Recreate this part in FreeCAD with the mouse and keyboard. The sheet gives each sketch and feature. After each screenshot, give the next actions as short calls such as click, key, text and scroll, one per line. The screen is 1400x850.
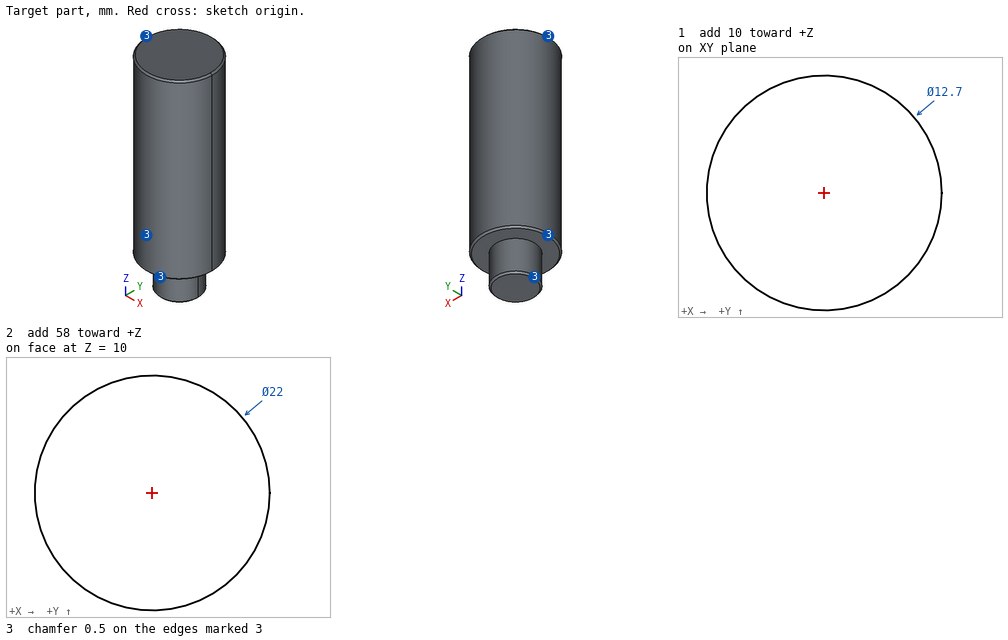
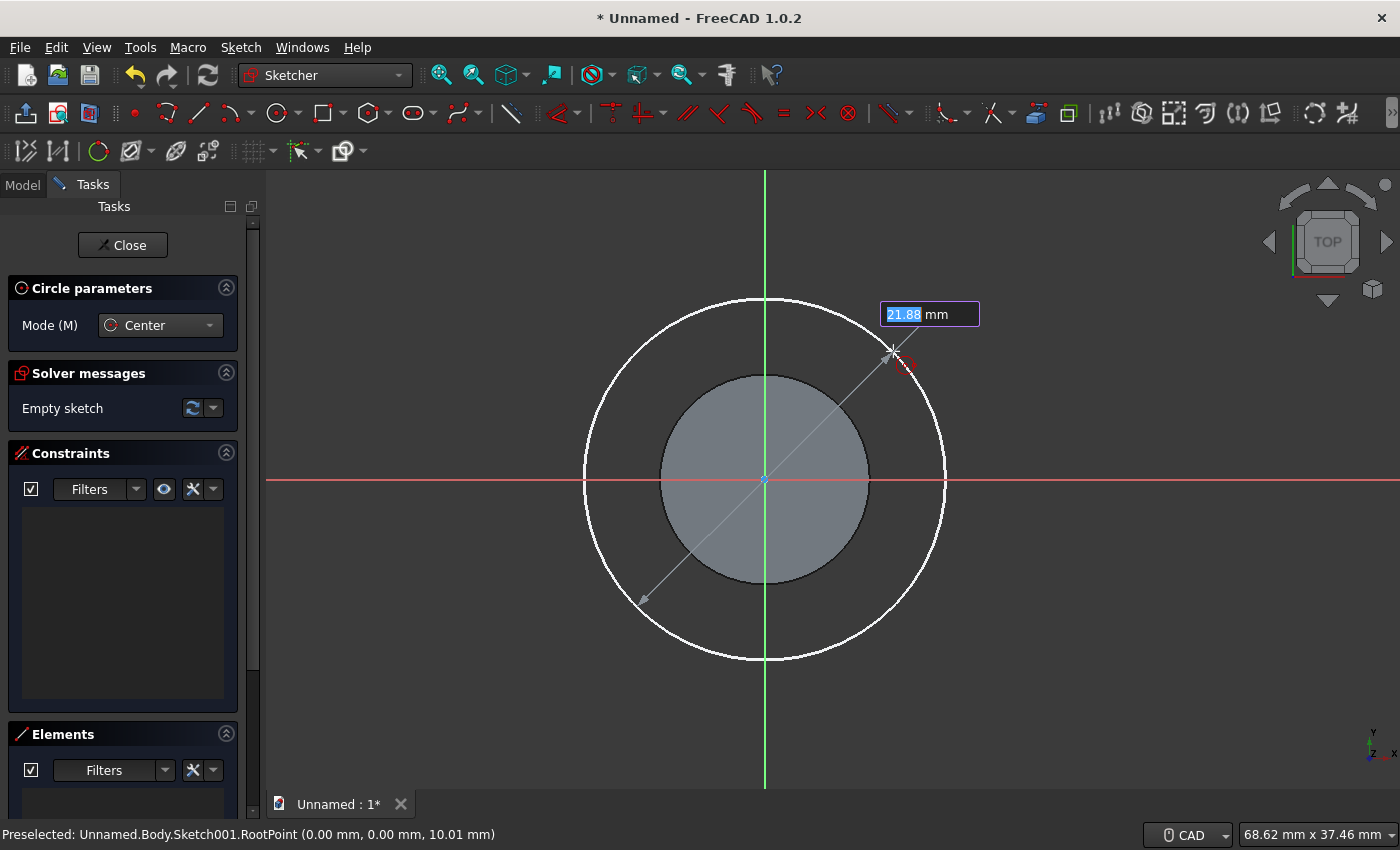
text(22)
key(Return)
key(Escape)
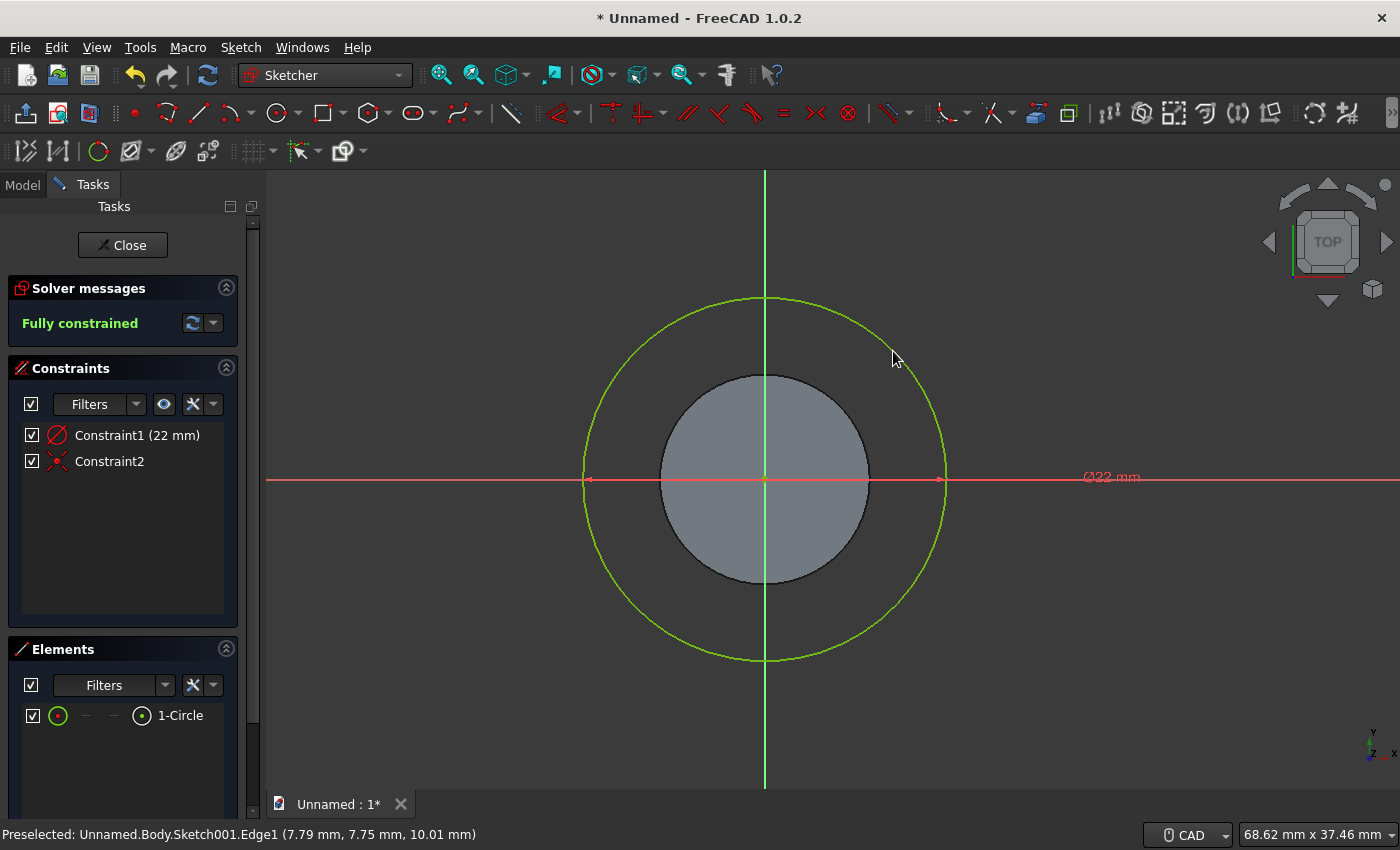
click(123, 245)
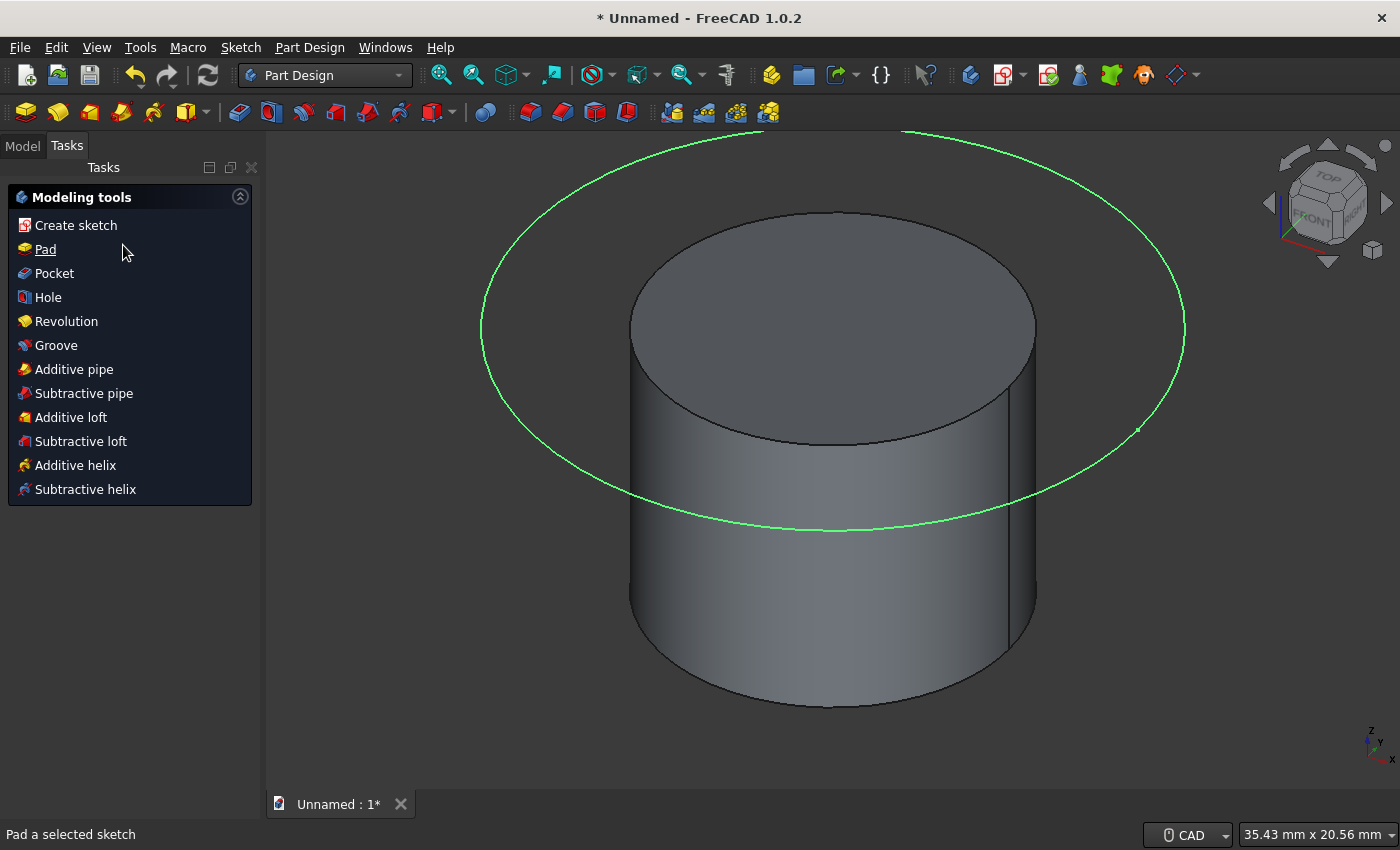
click(26, 112)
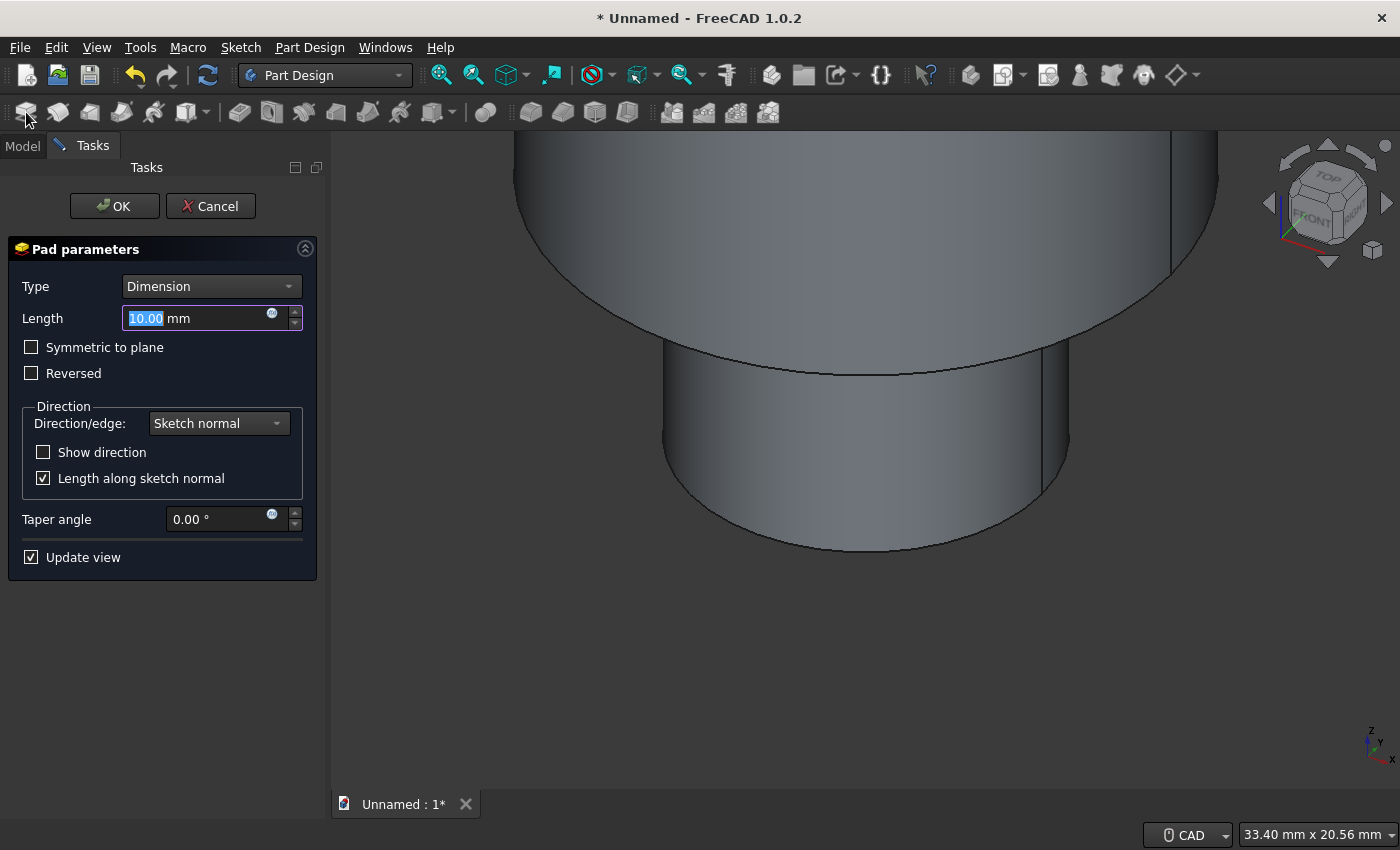
text(58)
key(Tab)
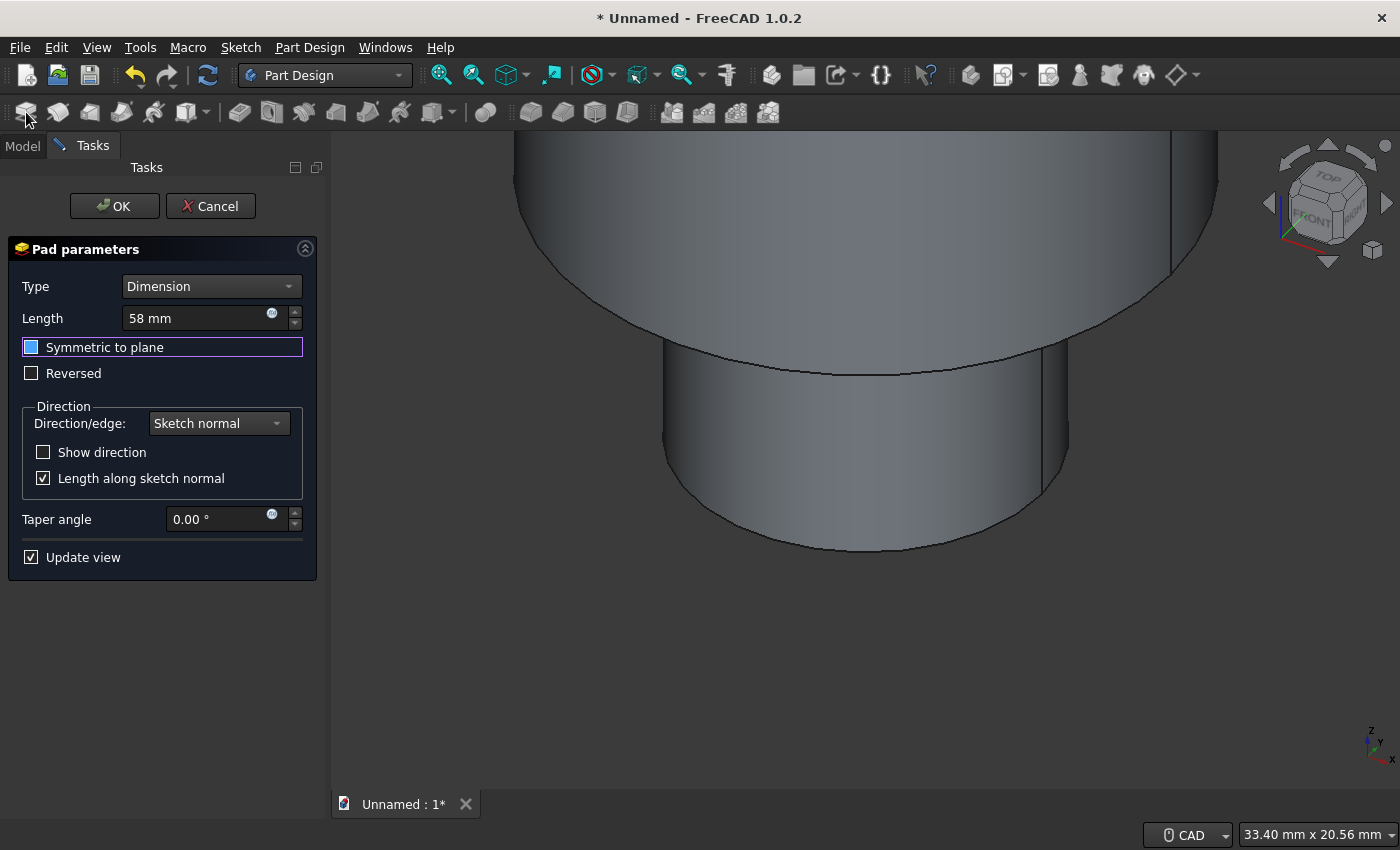
click(115, 206)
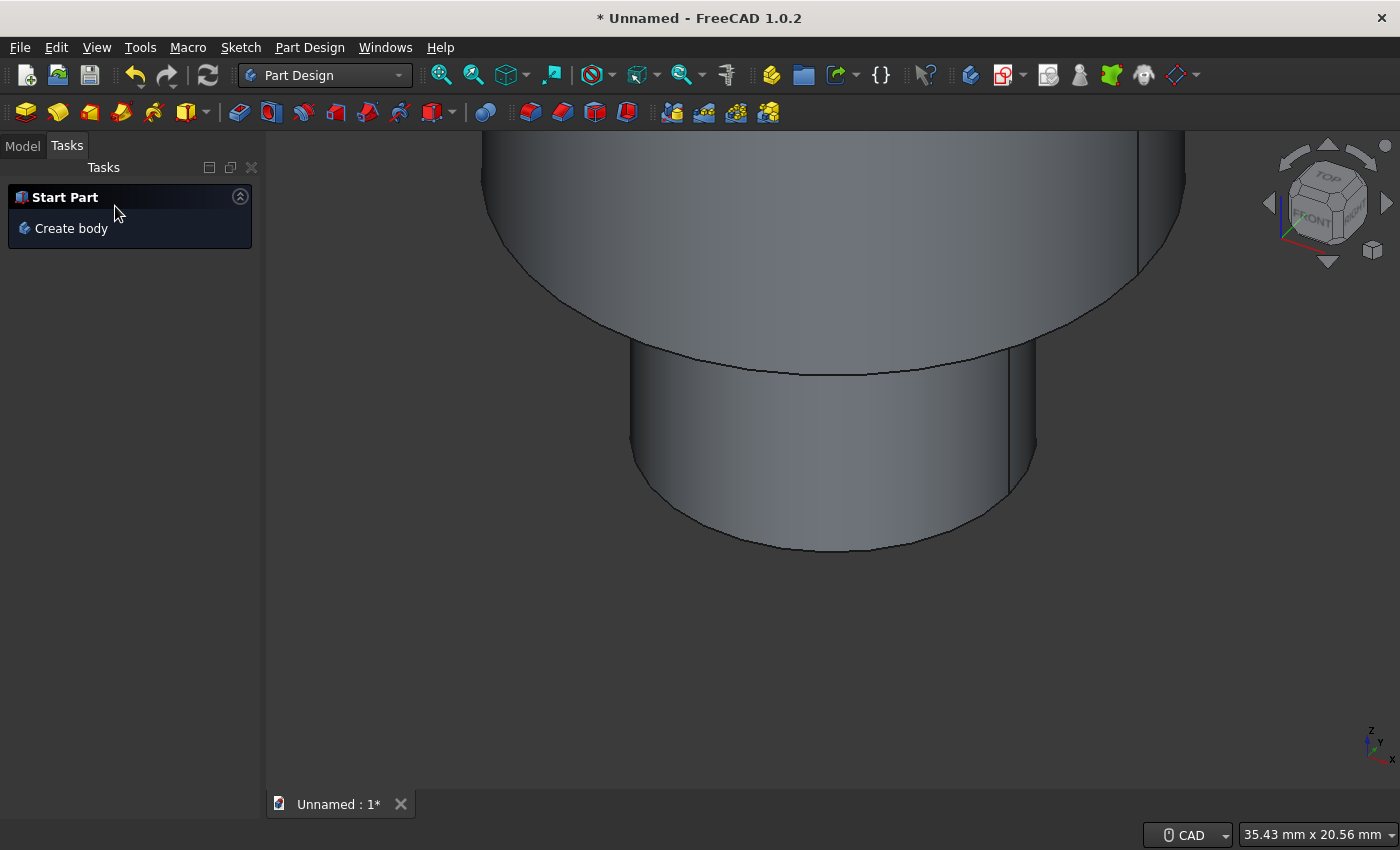
click(442, 76)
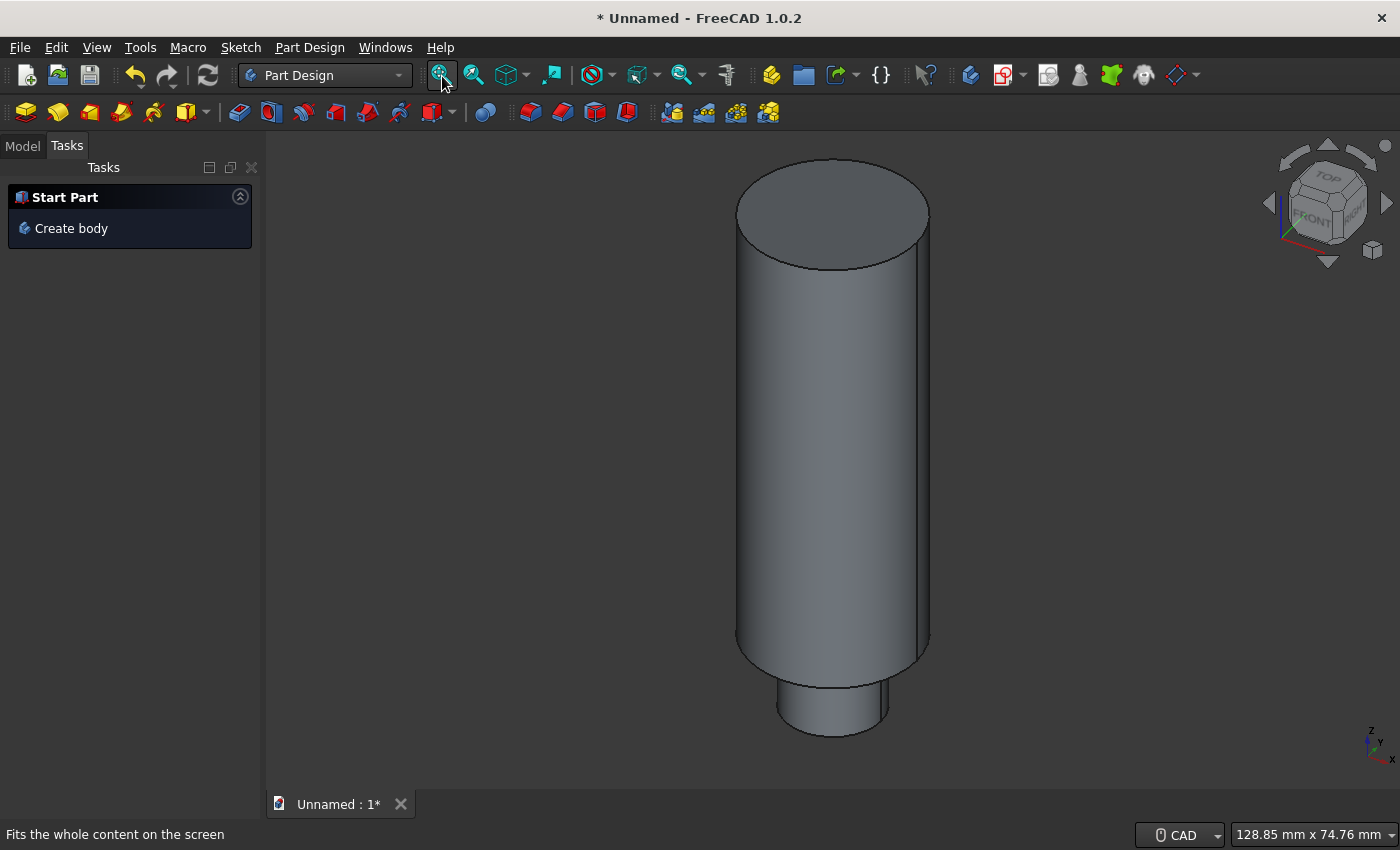
click(737, 220)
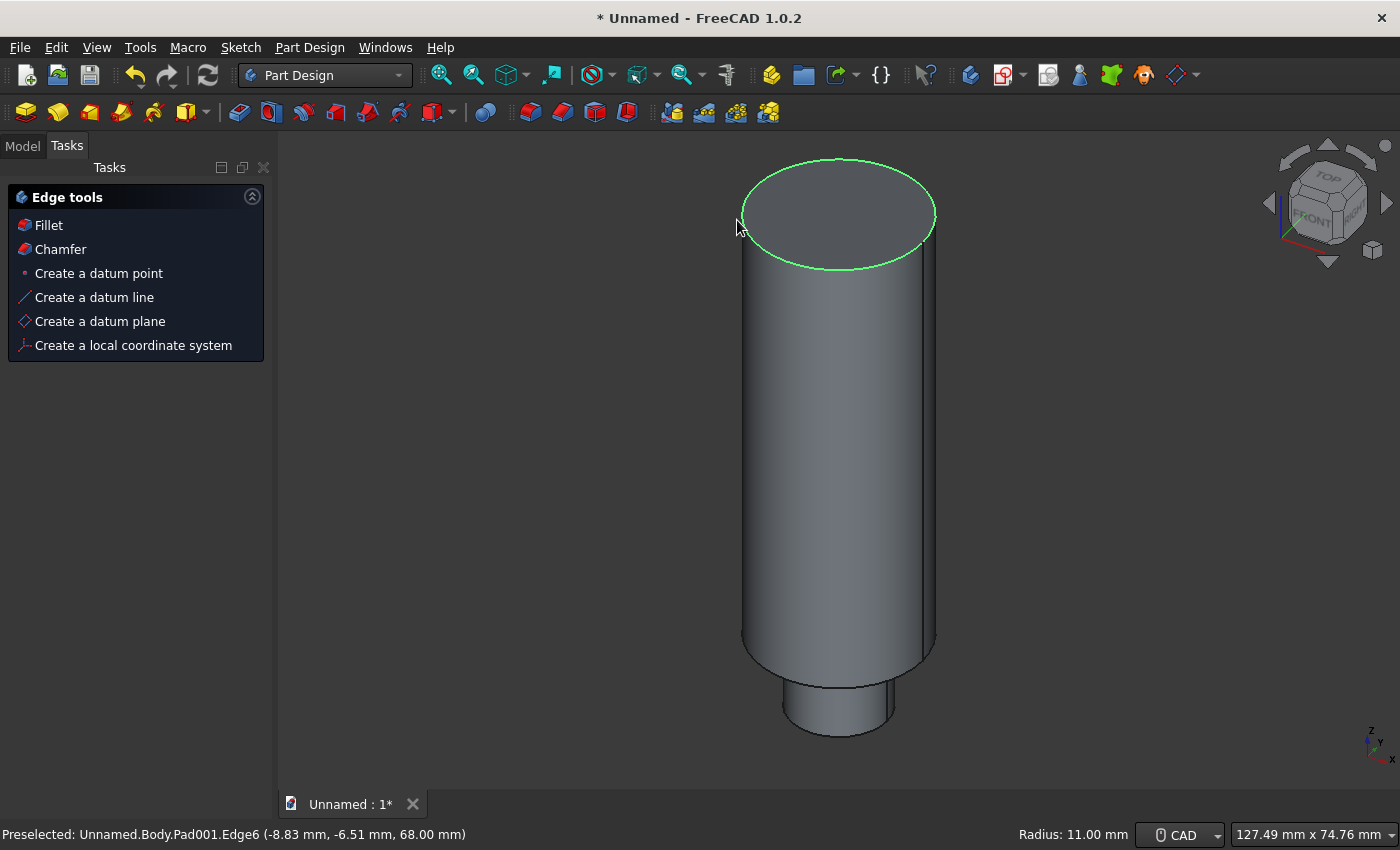
key(0)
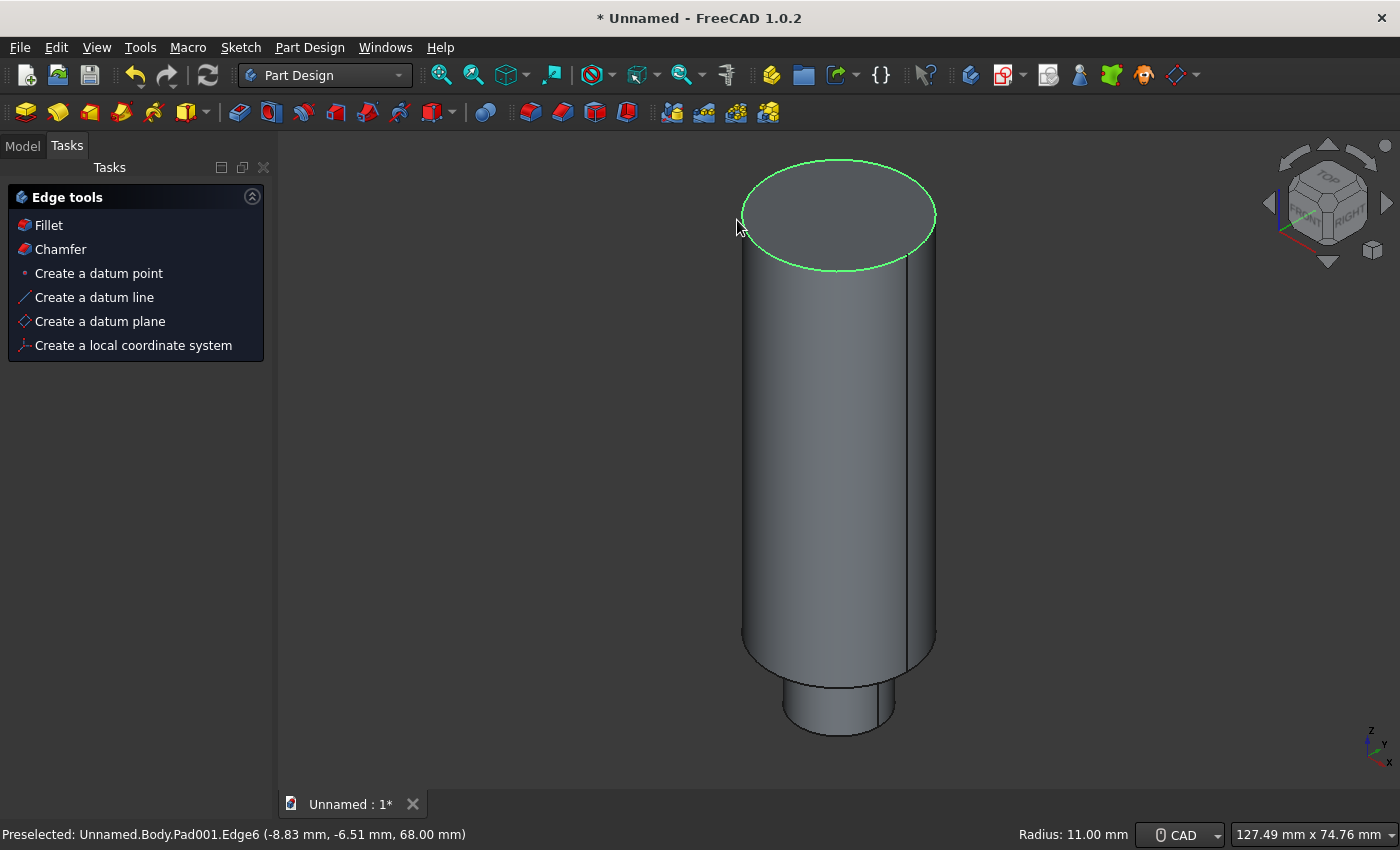
key(2)